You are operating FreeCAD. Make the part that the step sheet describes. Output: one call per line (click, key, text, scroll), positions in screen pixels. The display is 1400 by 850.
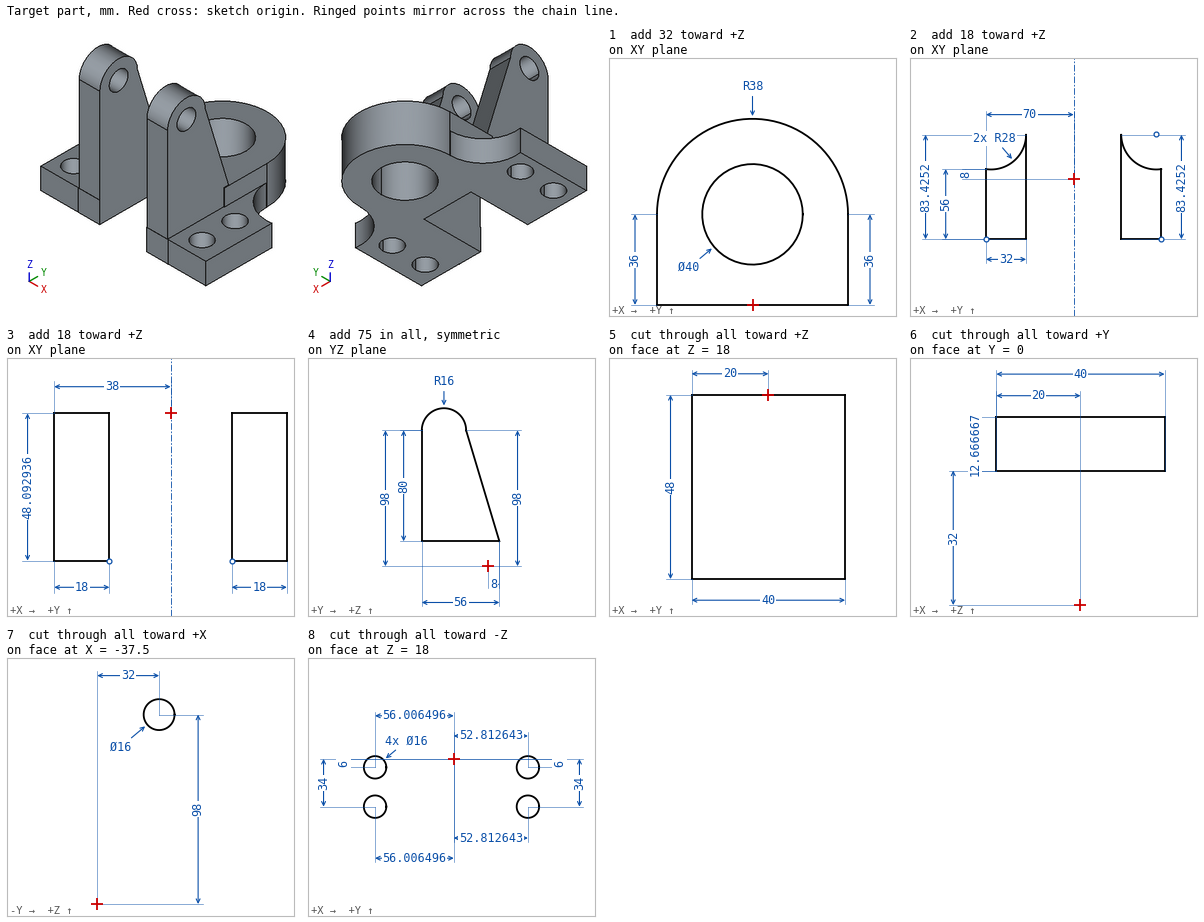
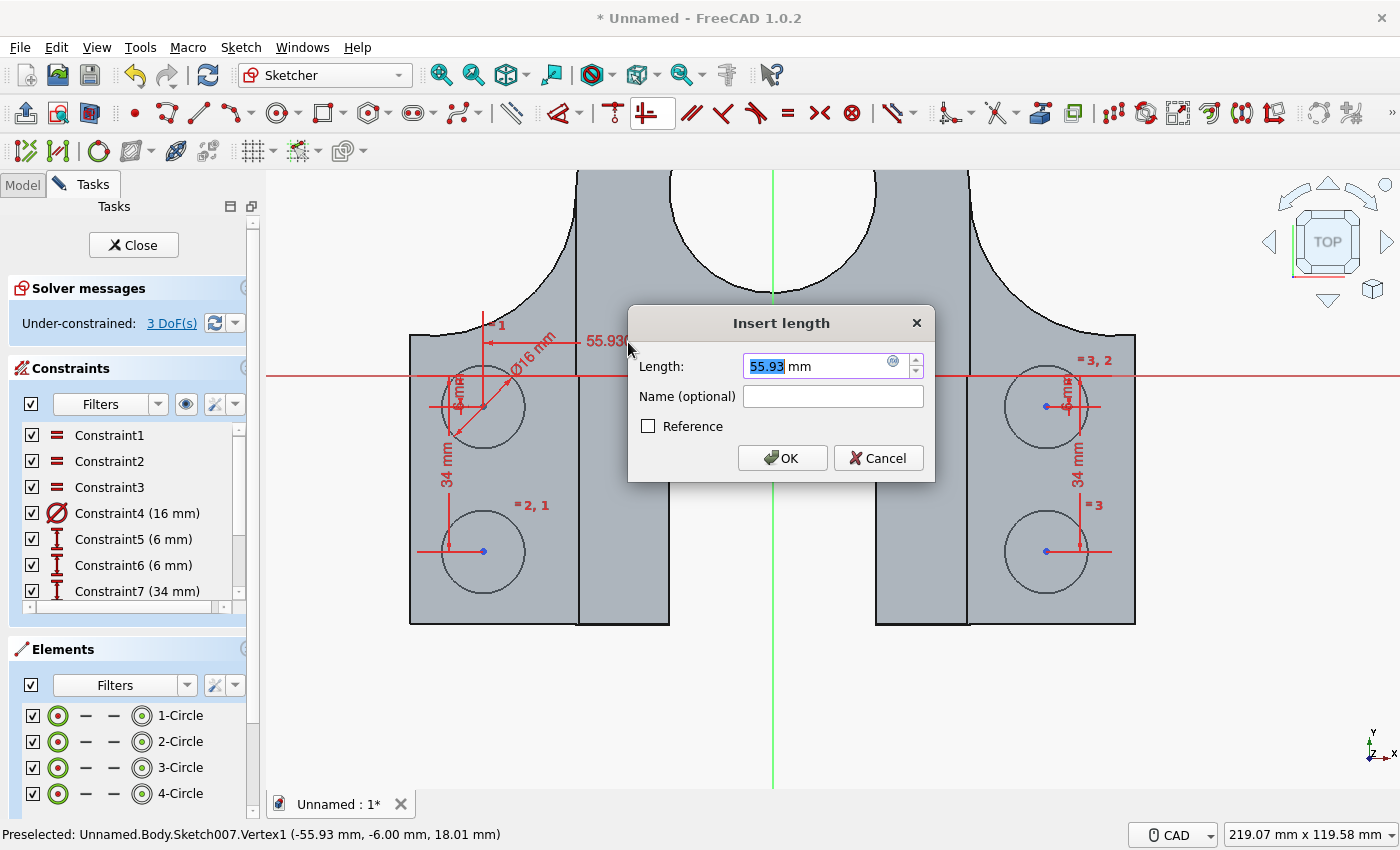
text(56.006496)
key(Return)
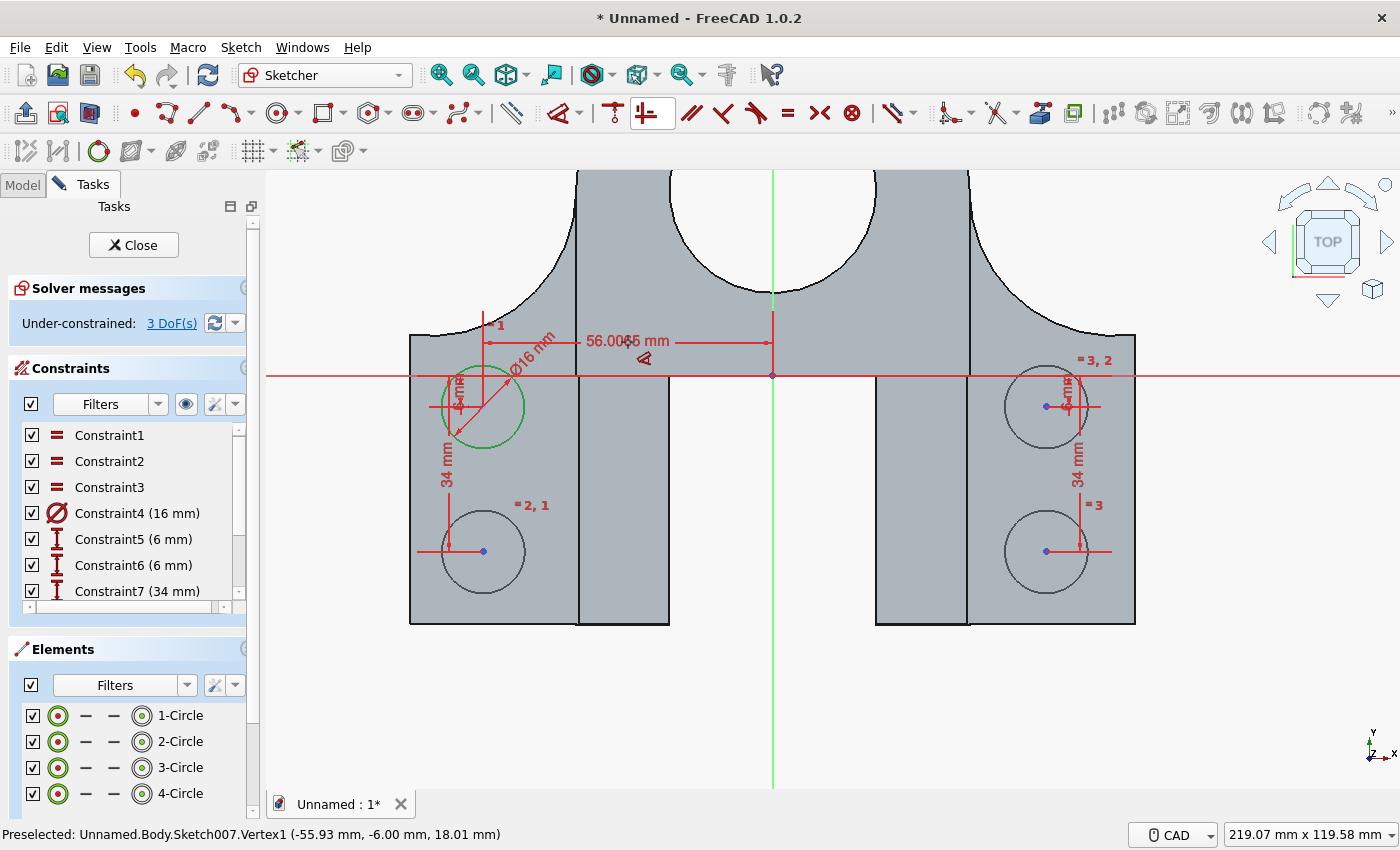
click(483, 552)
click(729, 342)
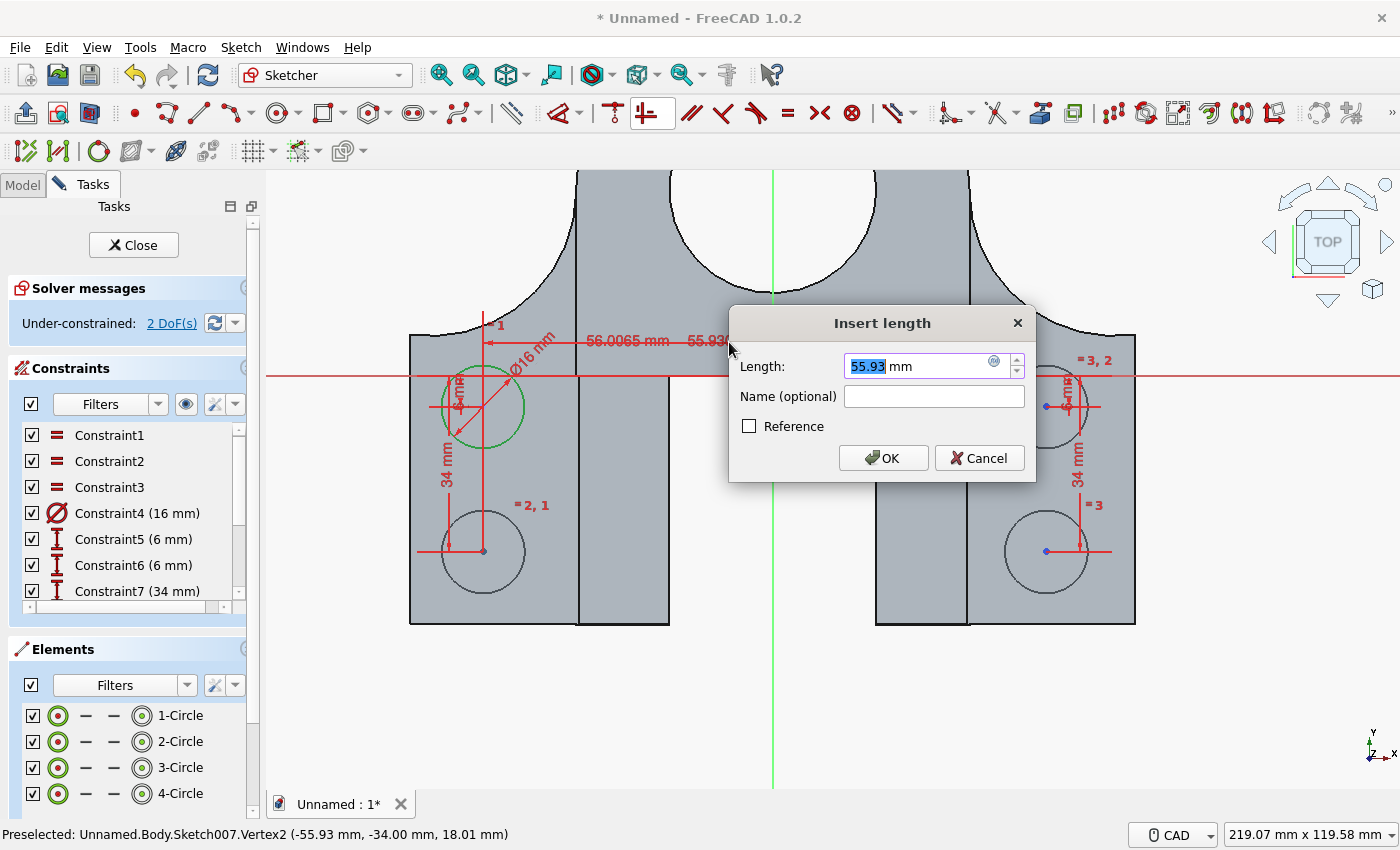
text(56.006496)
key(Return)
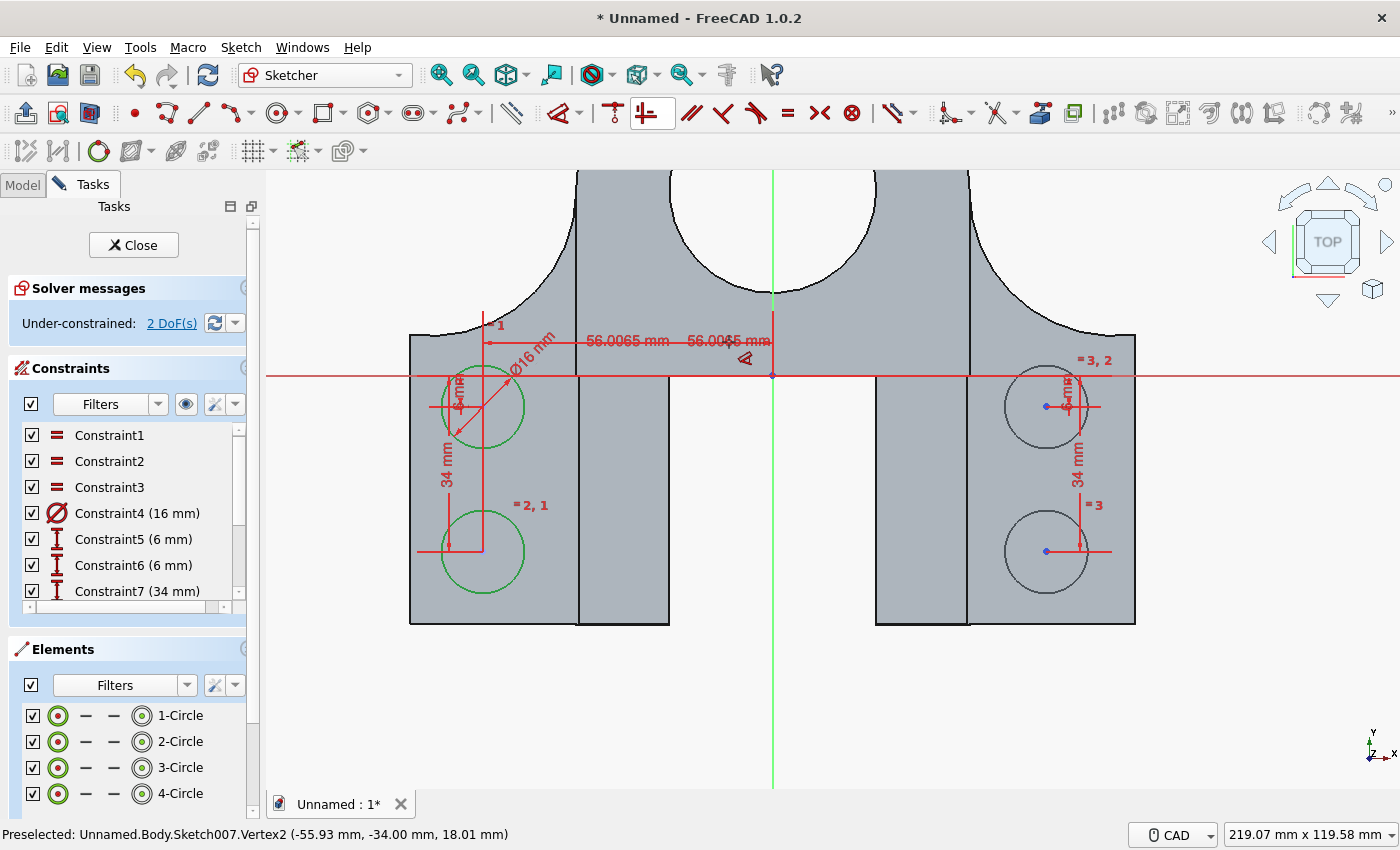
click(1046, 407)
click(910, 342)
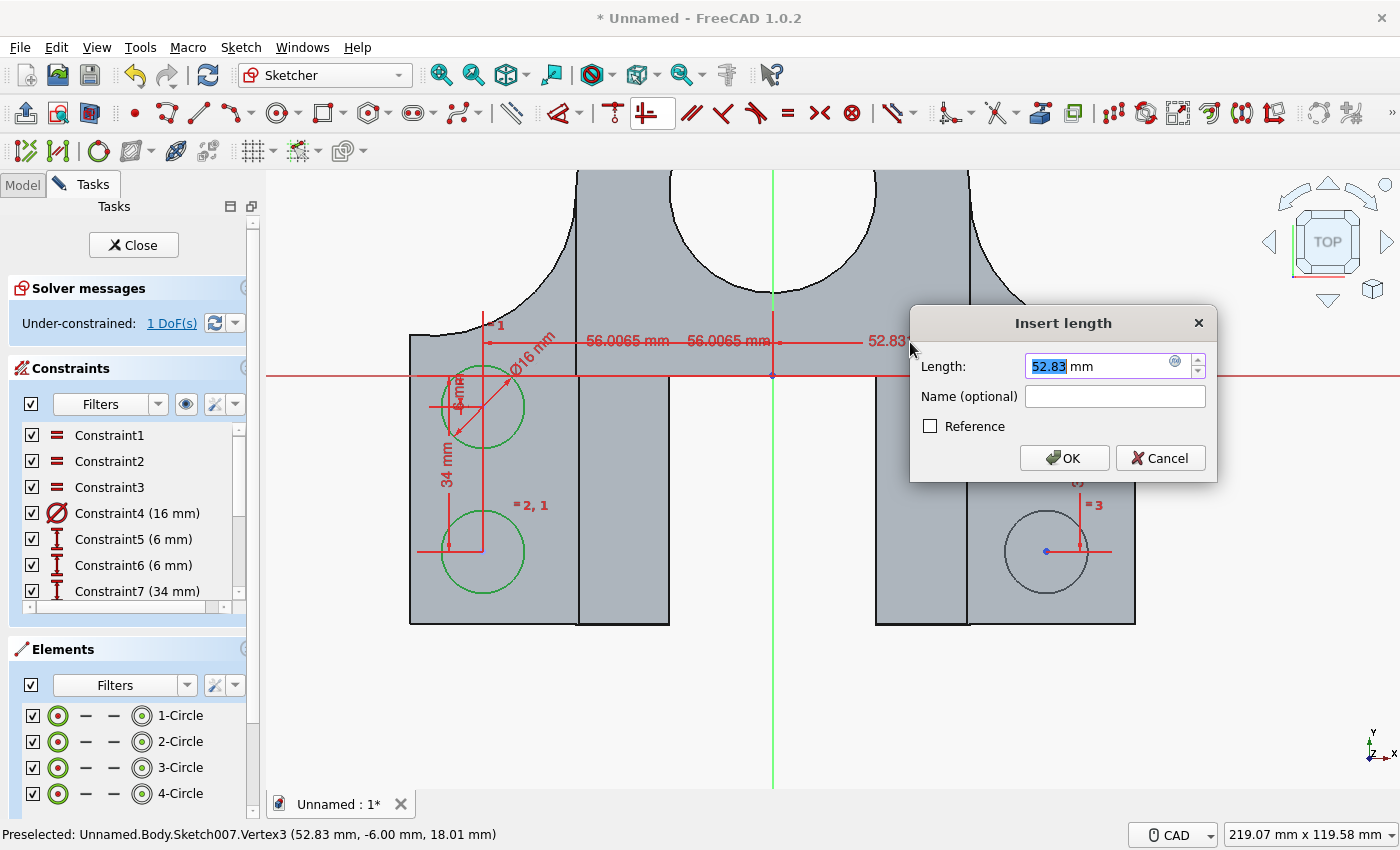
text(52.812643)
key(Return)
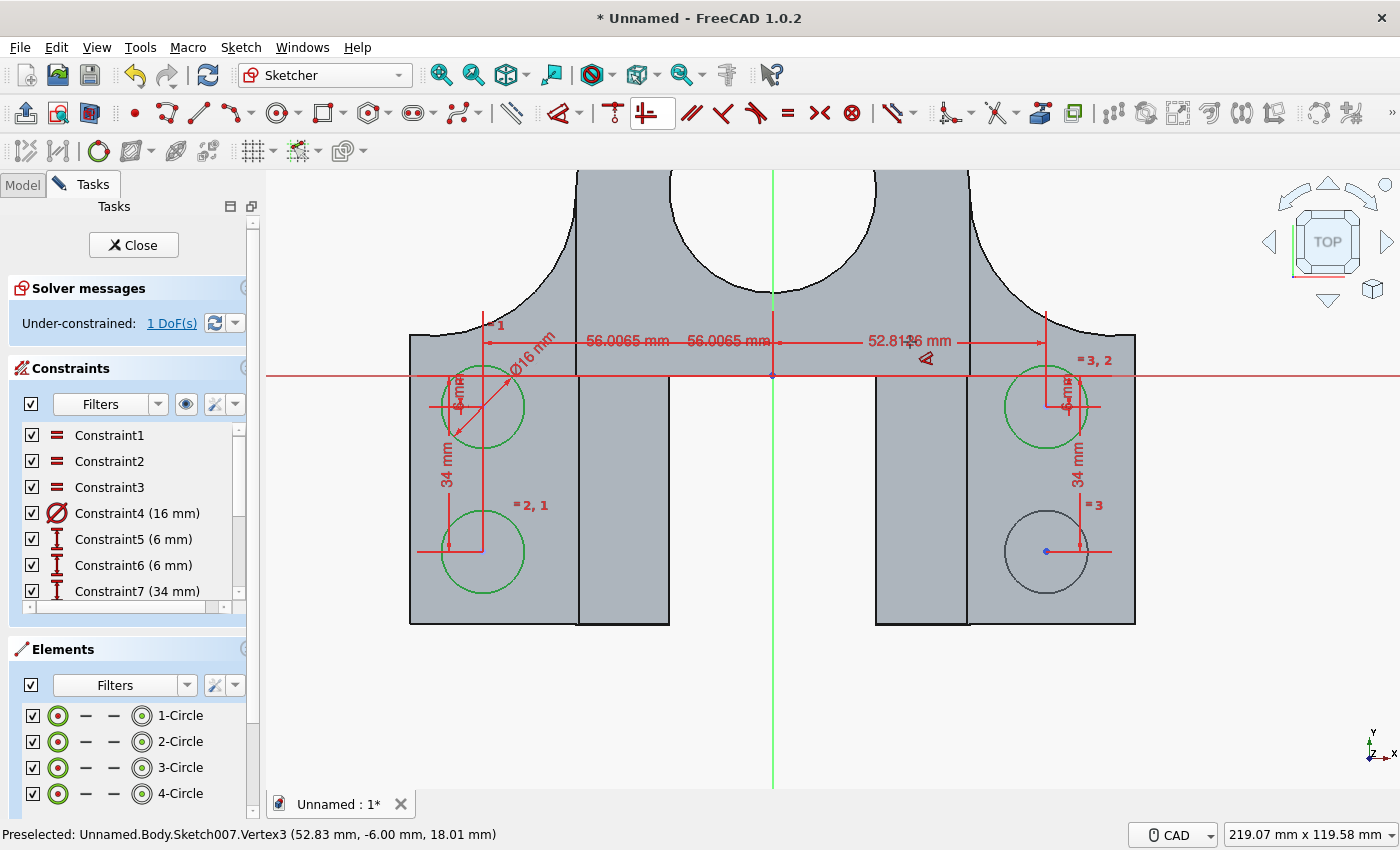
click(1046, 552)
click(814, 342)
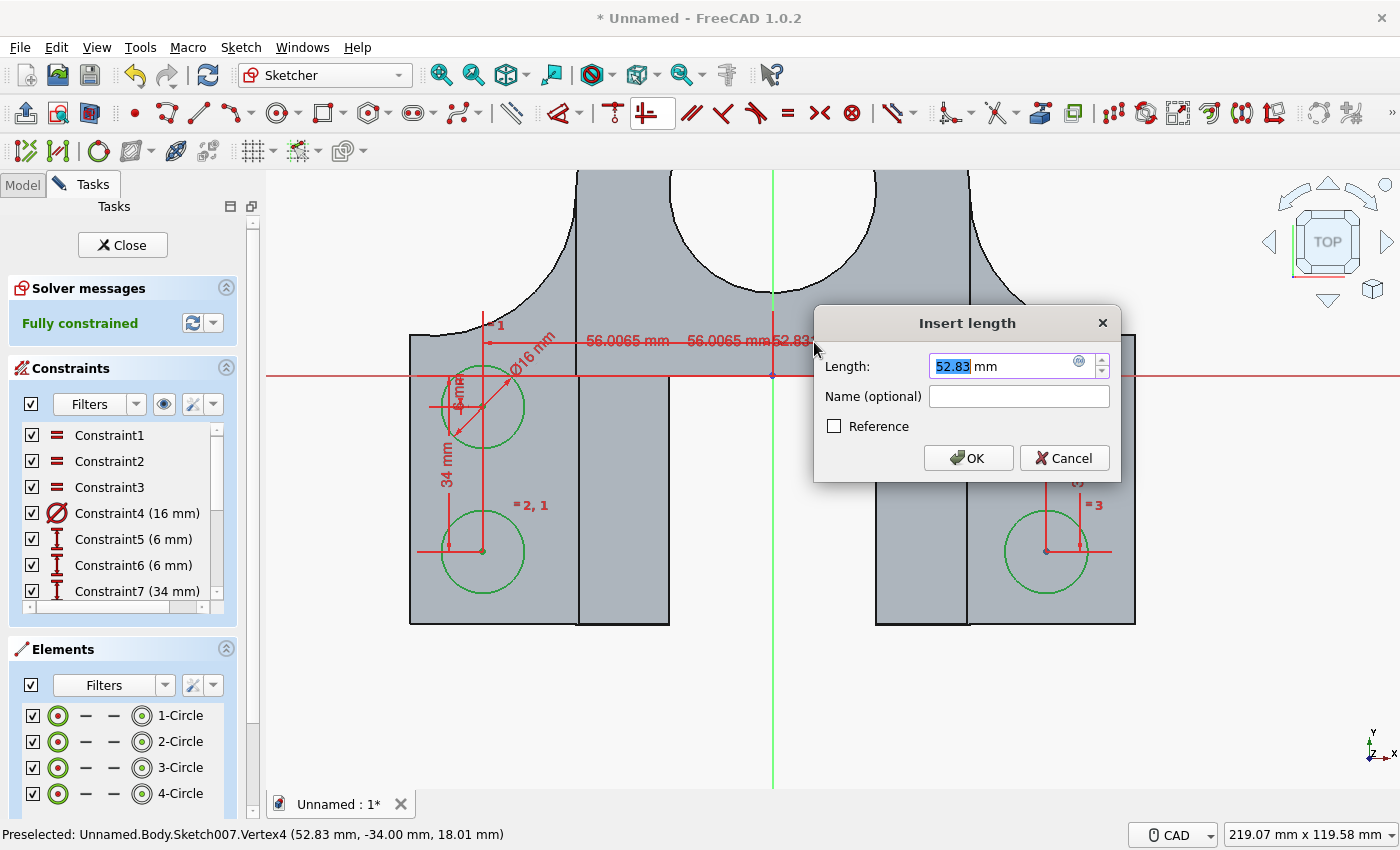
text(52.812643)
key(Return)
key(Escape)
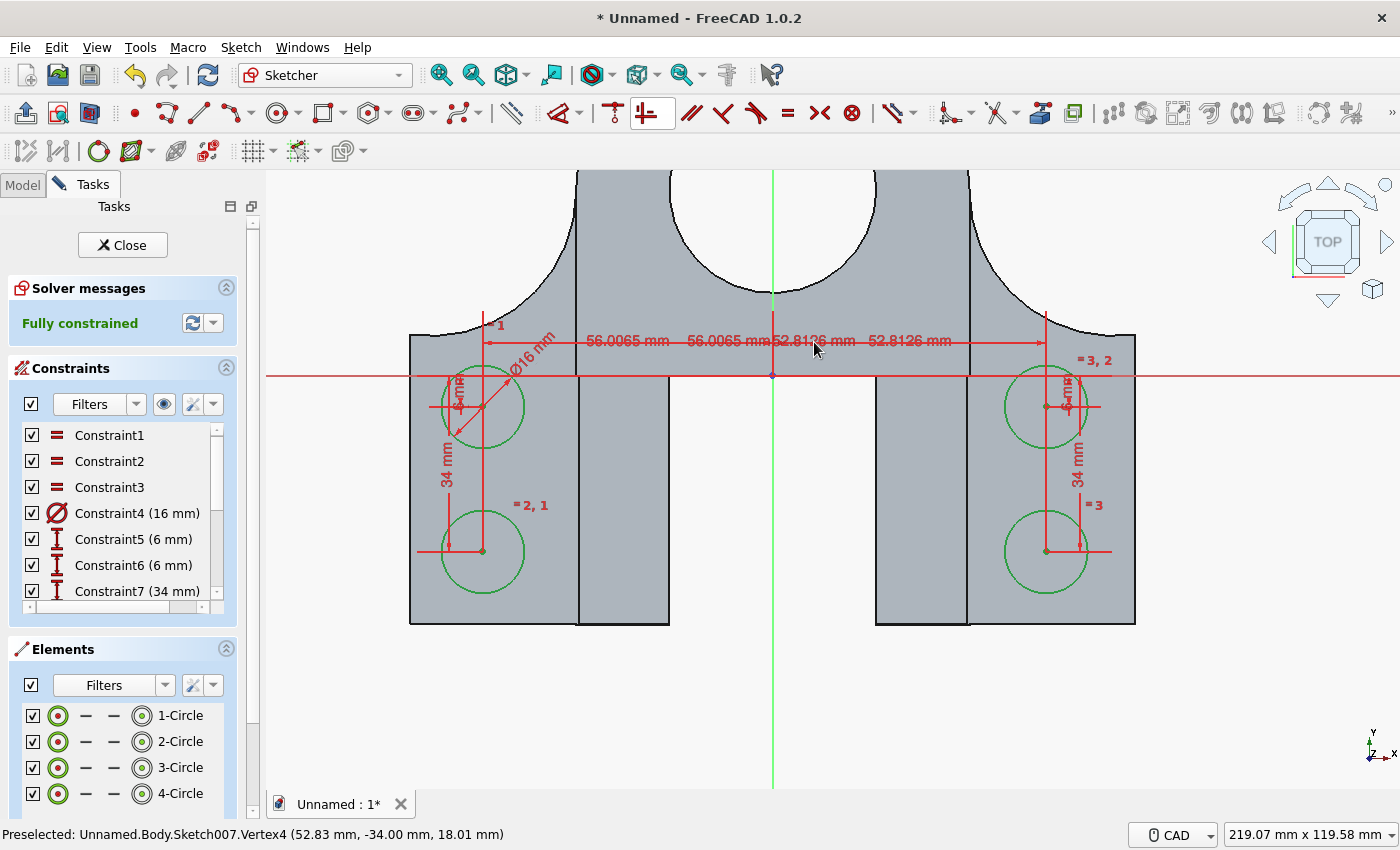
click(123, 245)